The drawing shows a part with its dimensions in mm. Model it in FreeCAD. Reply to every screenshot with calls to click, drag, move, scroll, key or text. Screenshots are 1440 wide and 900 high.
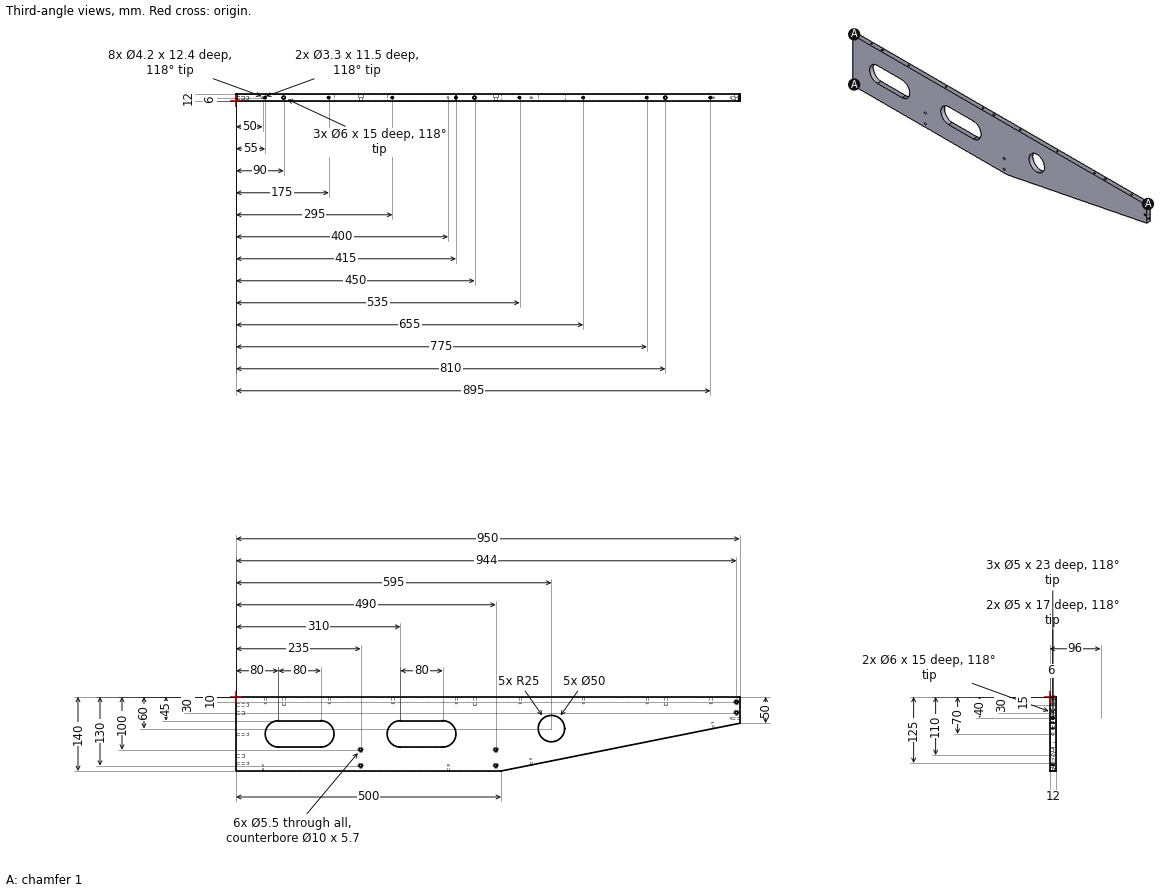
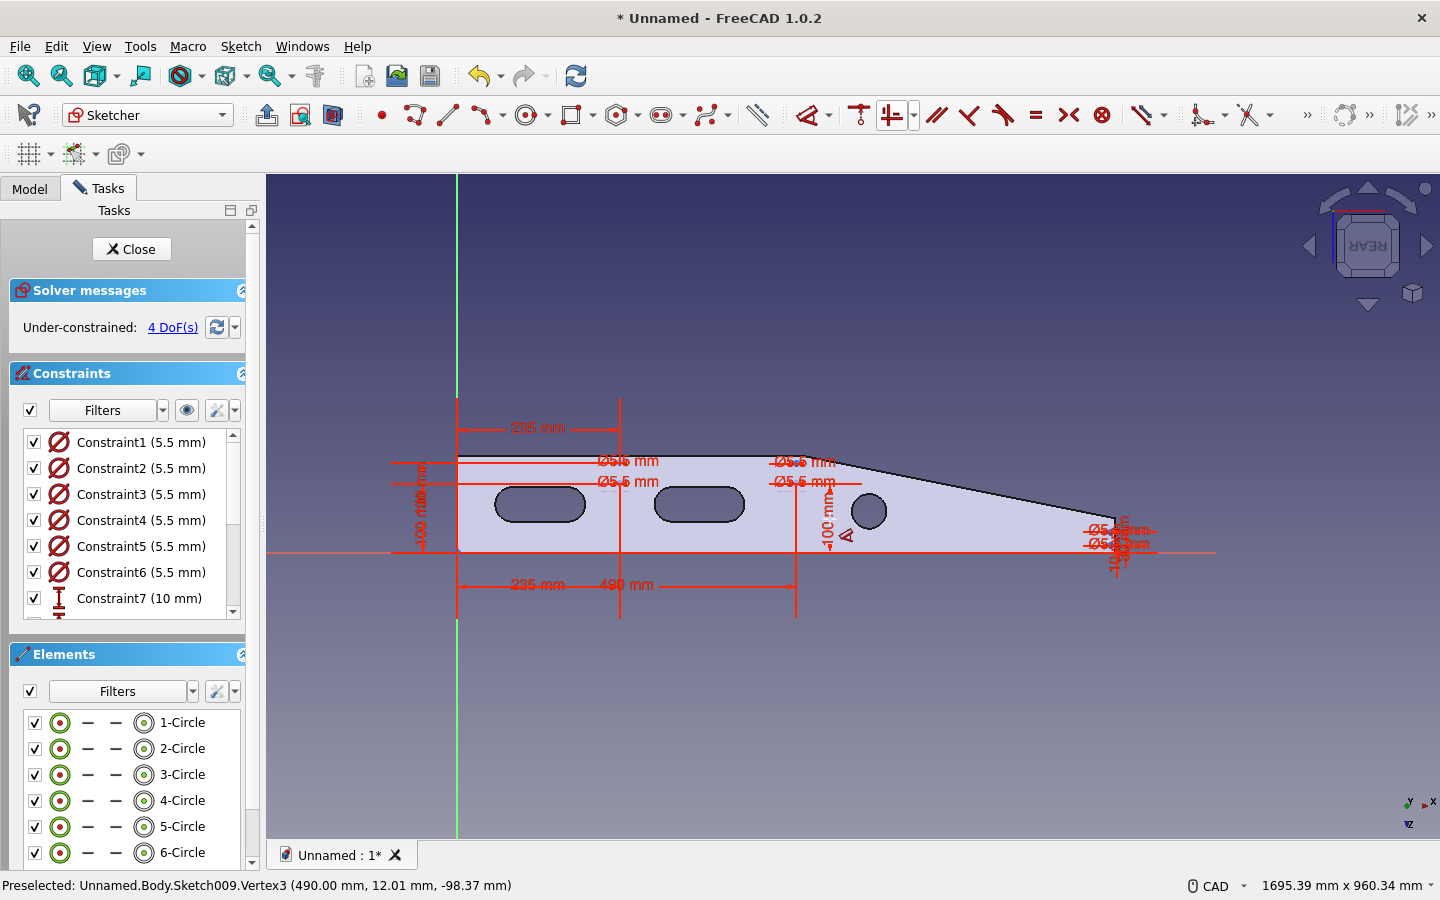
click(797, 464)
click(705, 587)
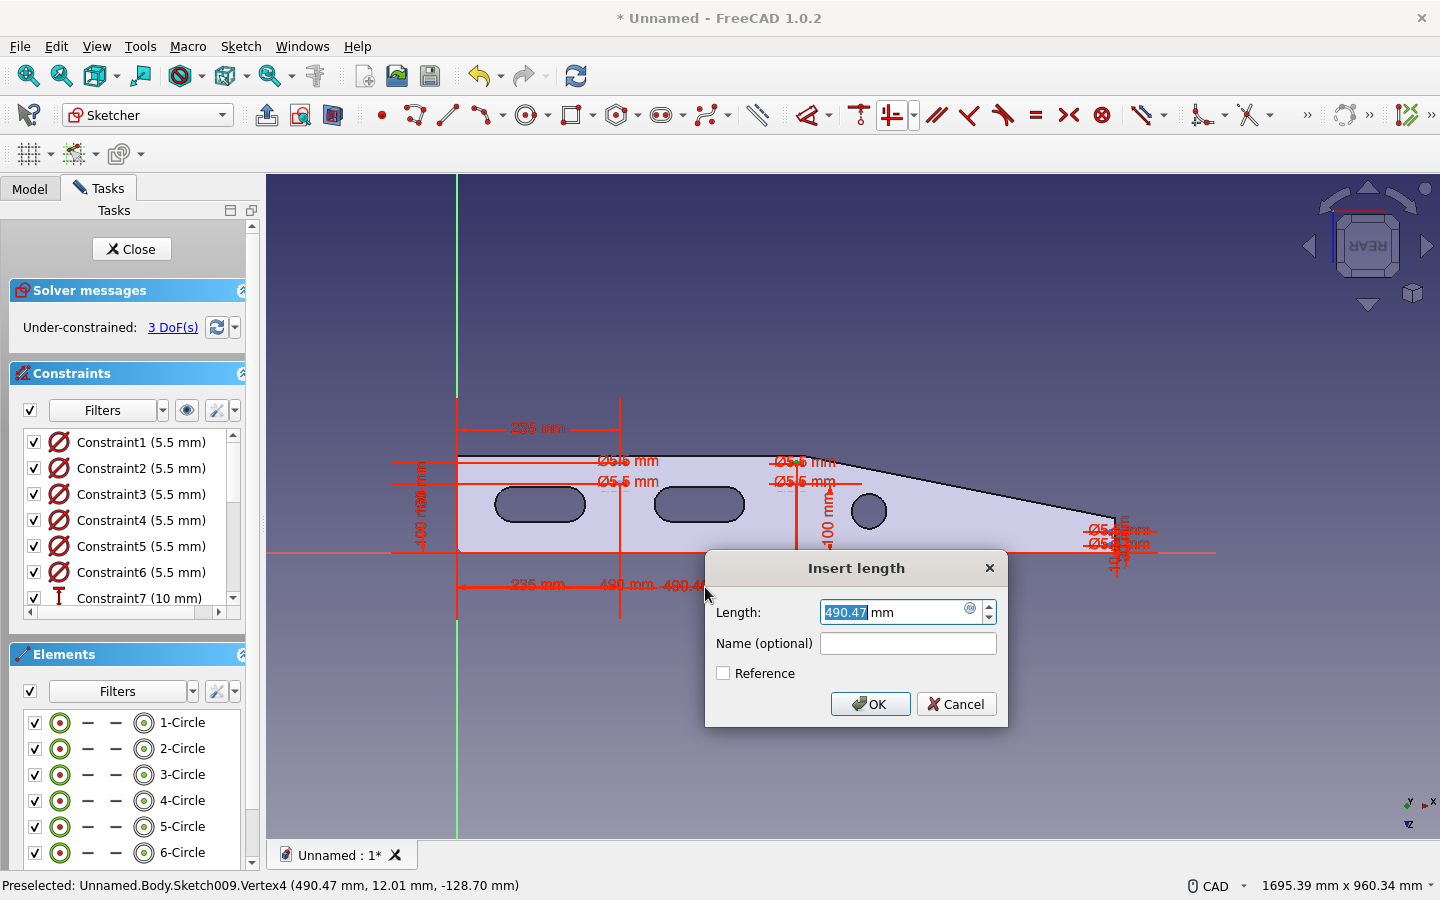
text(490)
key(Return)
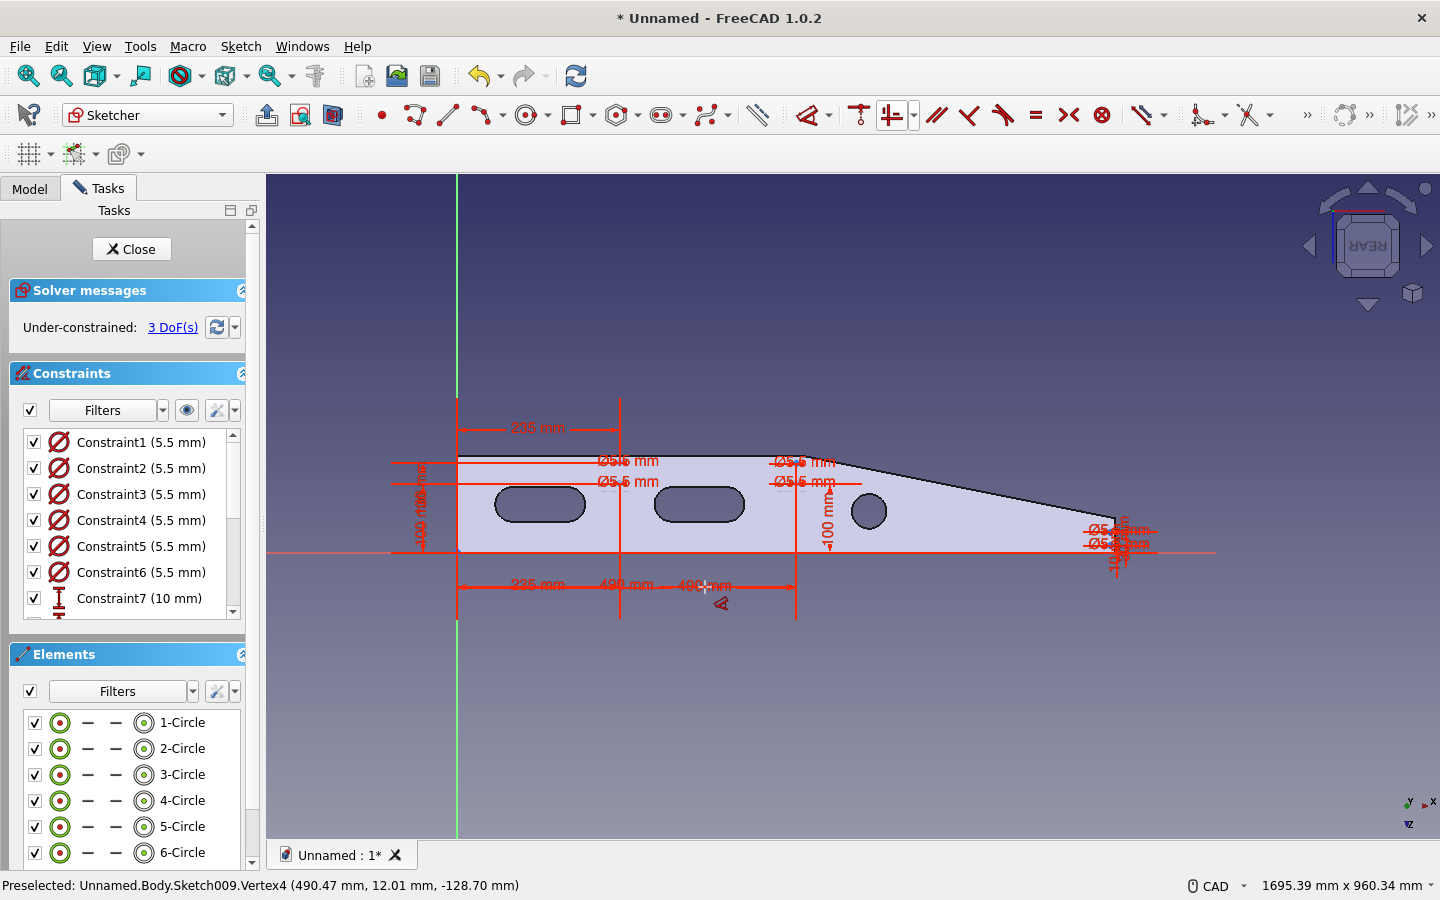
click(796, 464)
click(423, 540)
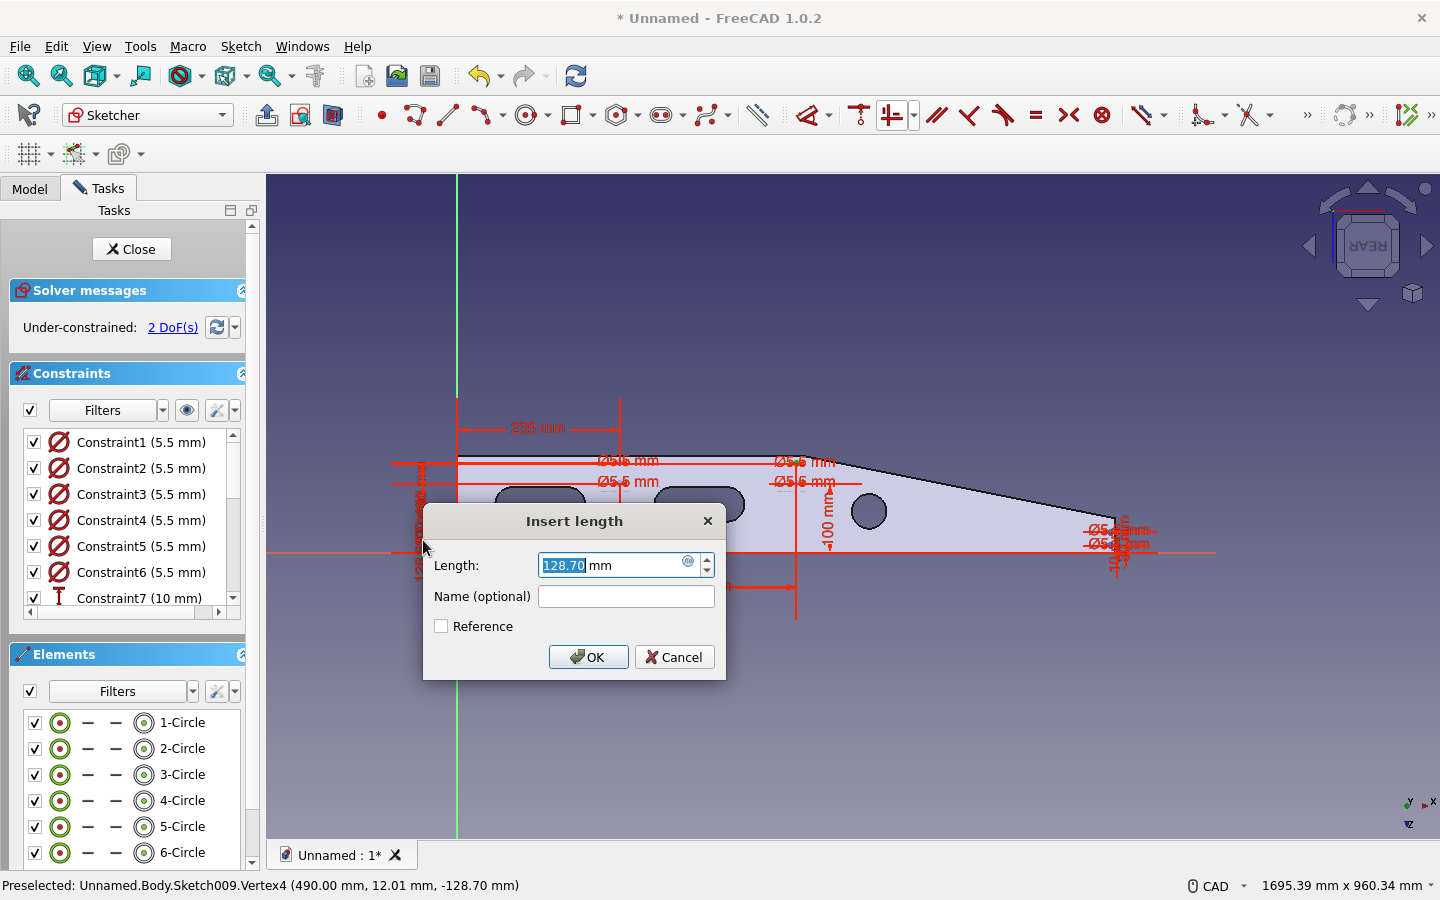
text(130)
key(Return)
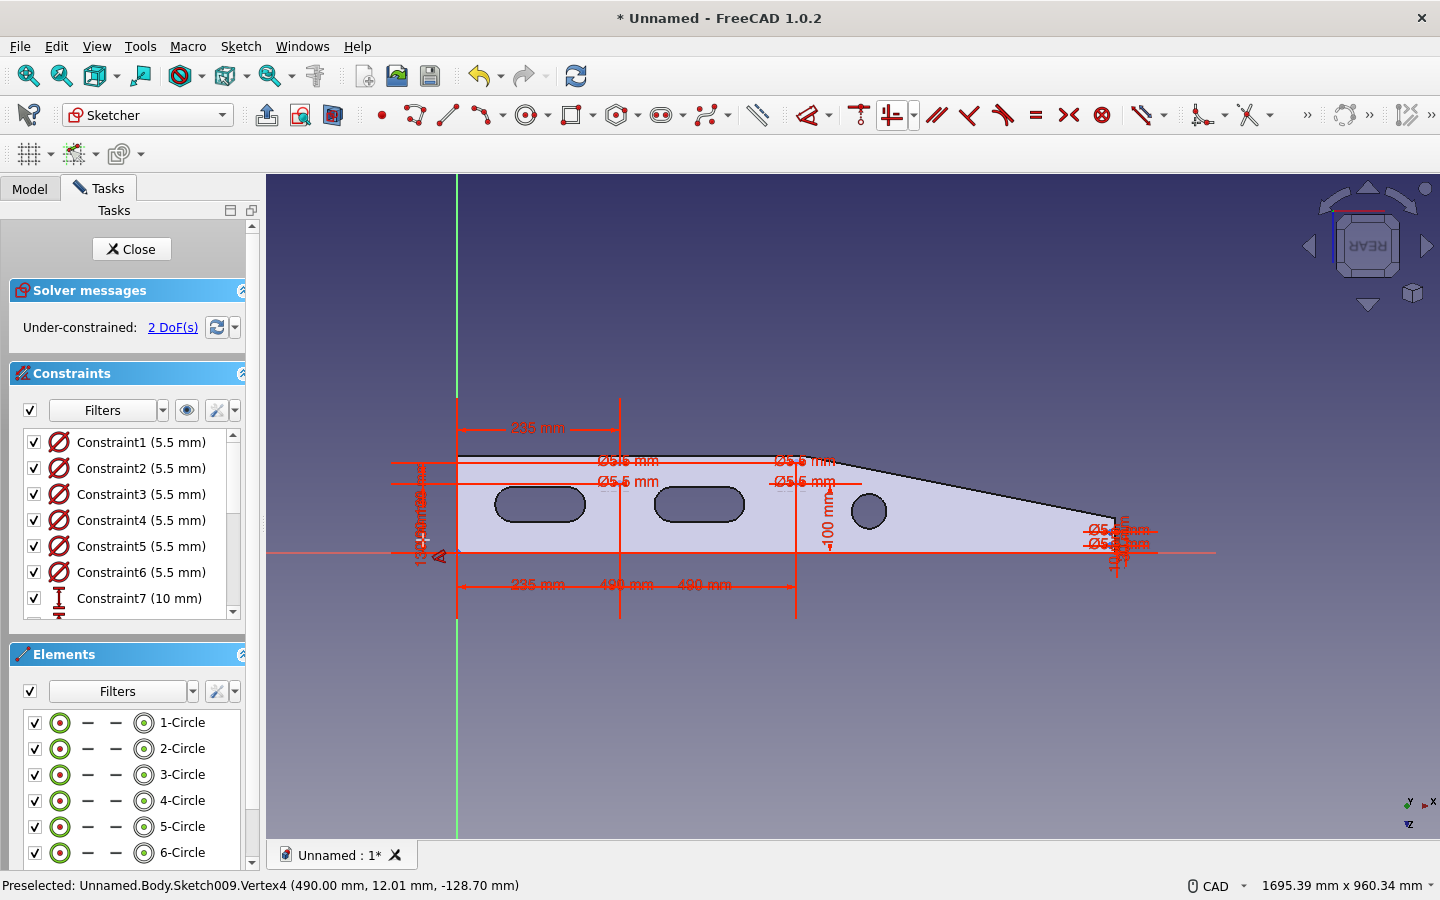
click(1111, 546)
click(784, 587)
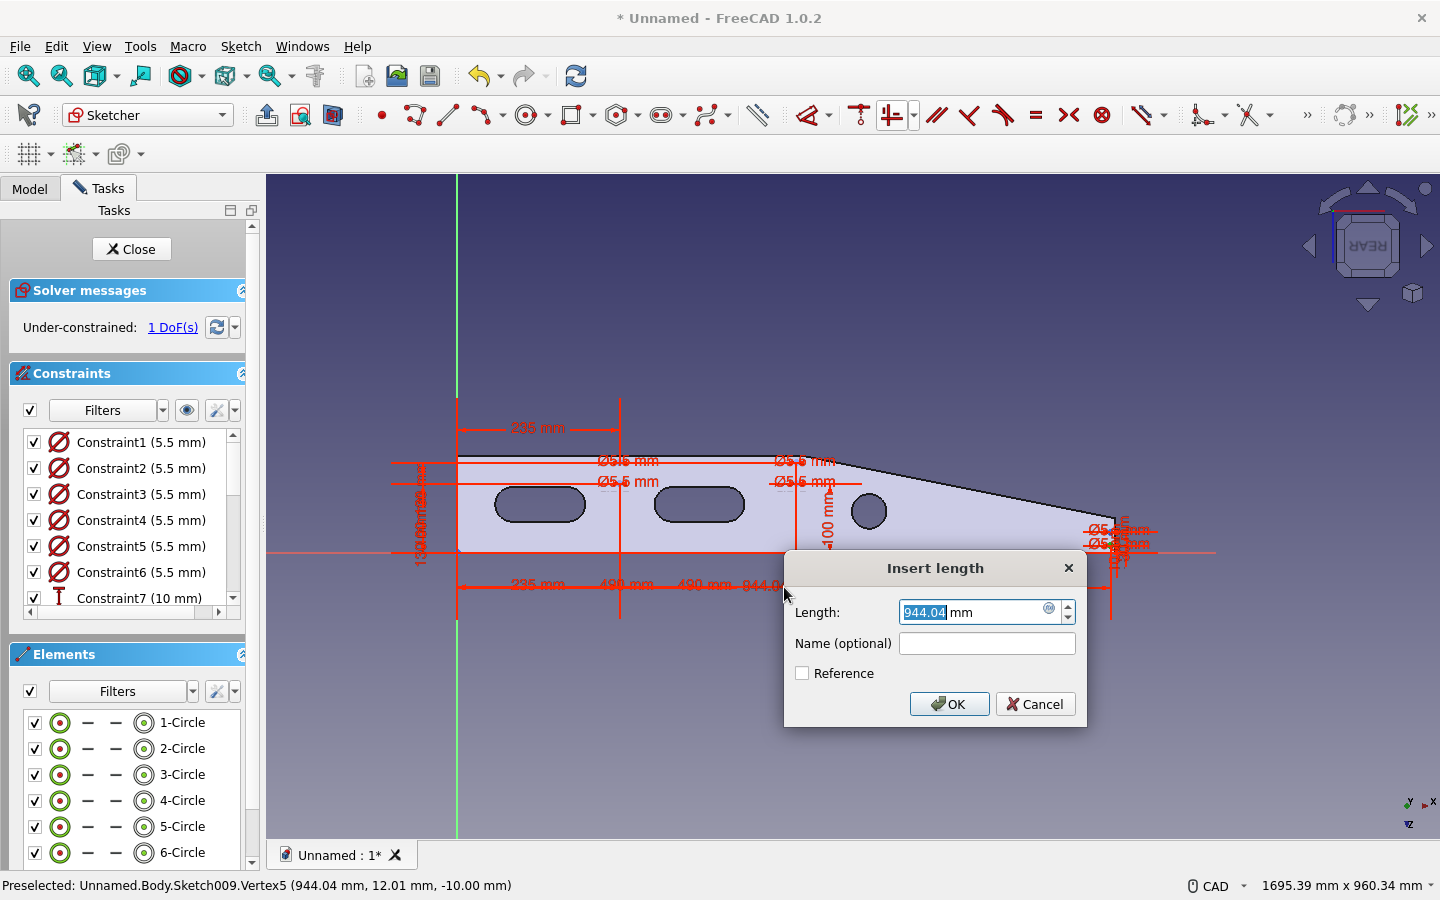
text(944)
key(Return)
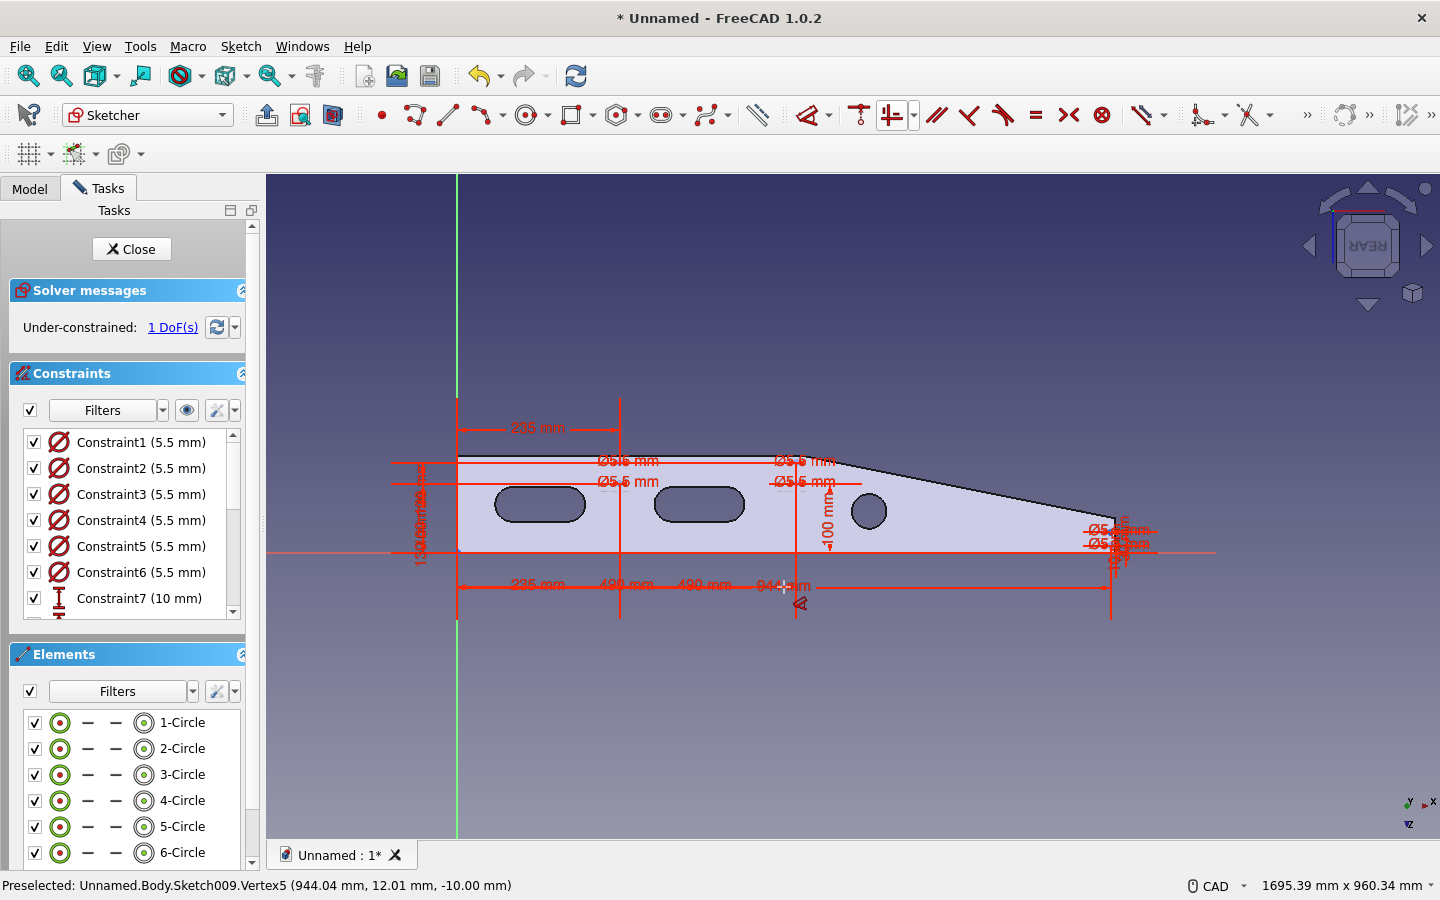
click(1111, 532)
click(934, 587)